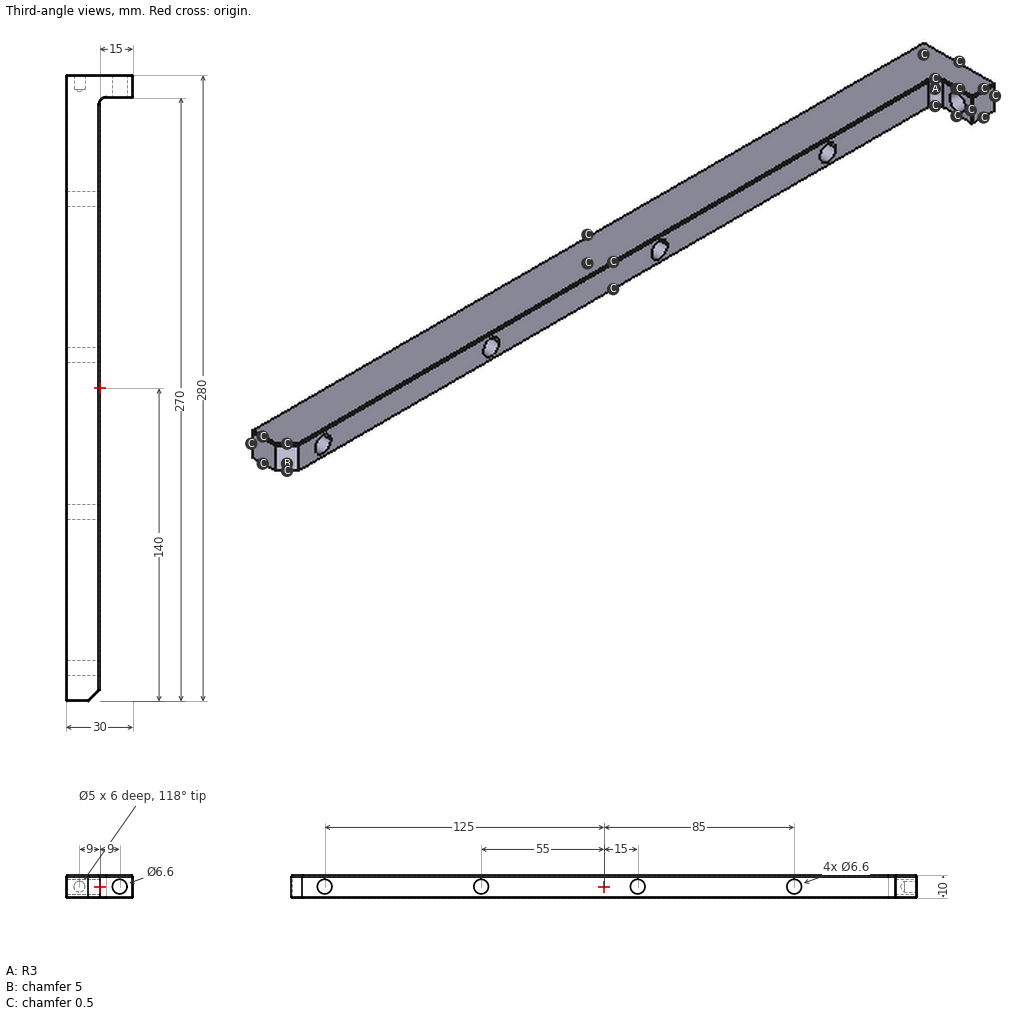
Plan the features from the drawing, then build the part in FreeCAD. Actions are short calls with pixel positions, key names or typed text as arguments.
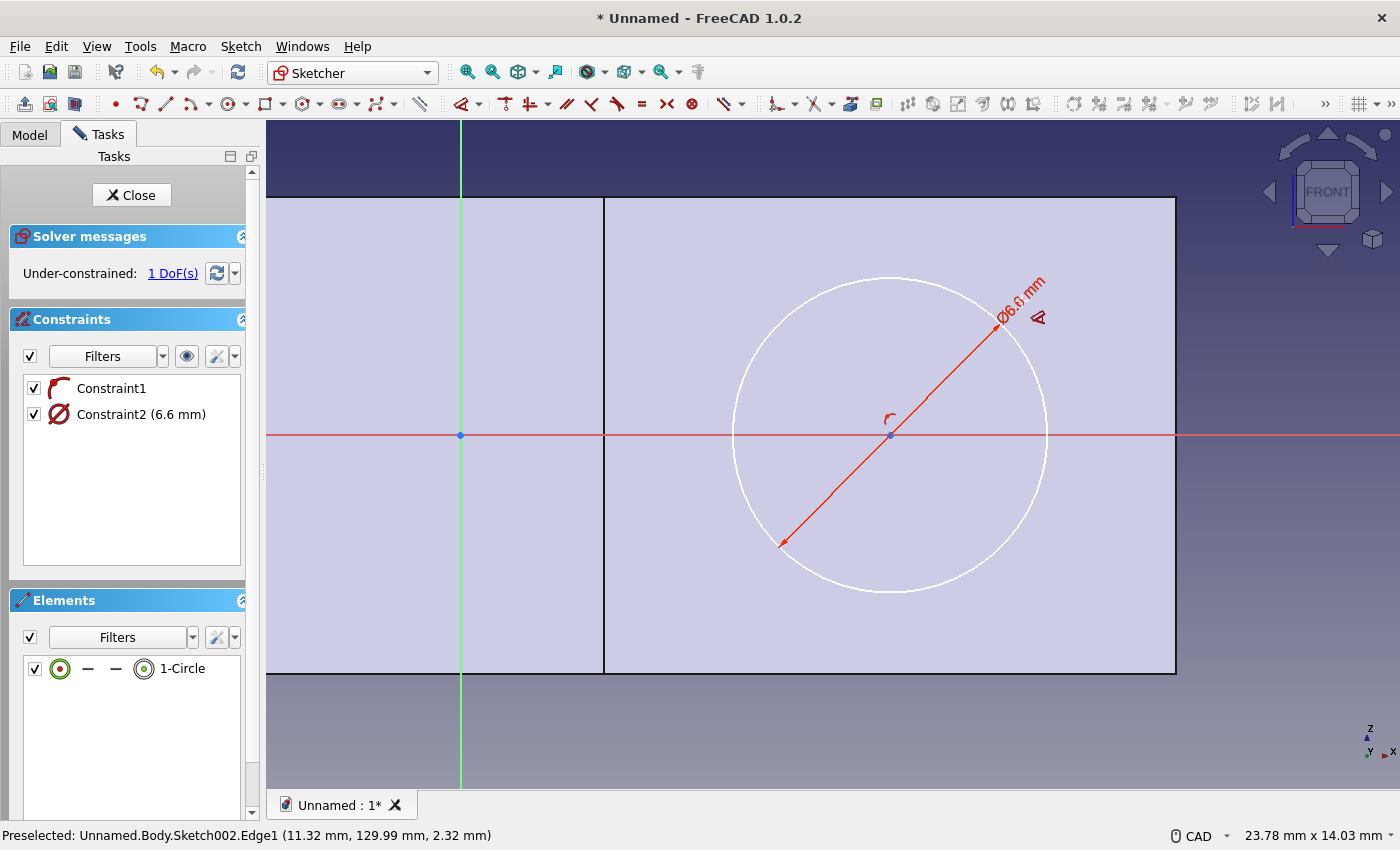
click(890, 435)
click(675, 469)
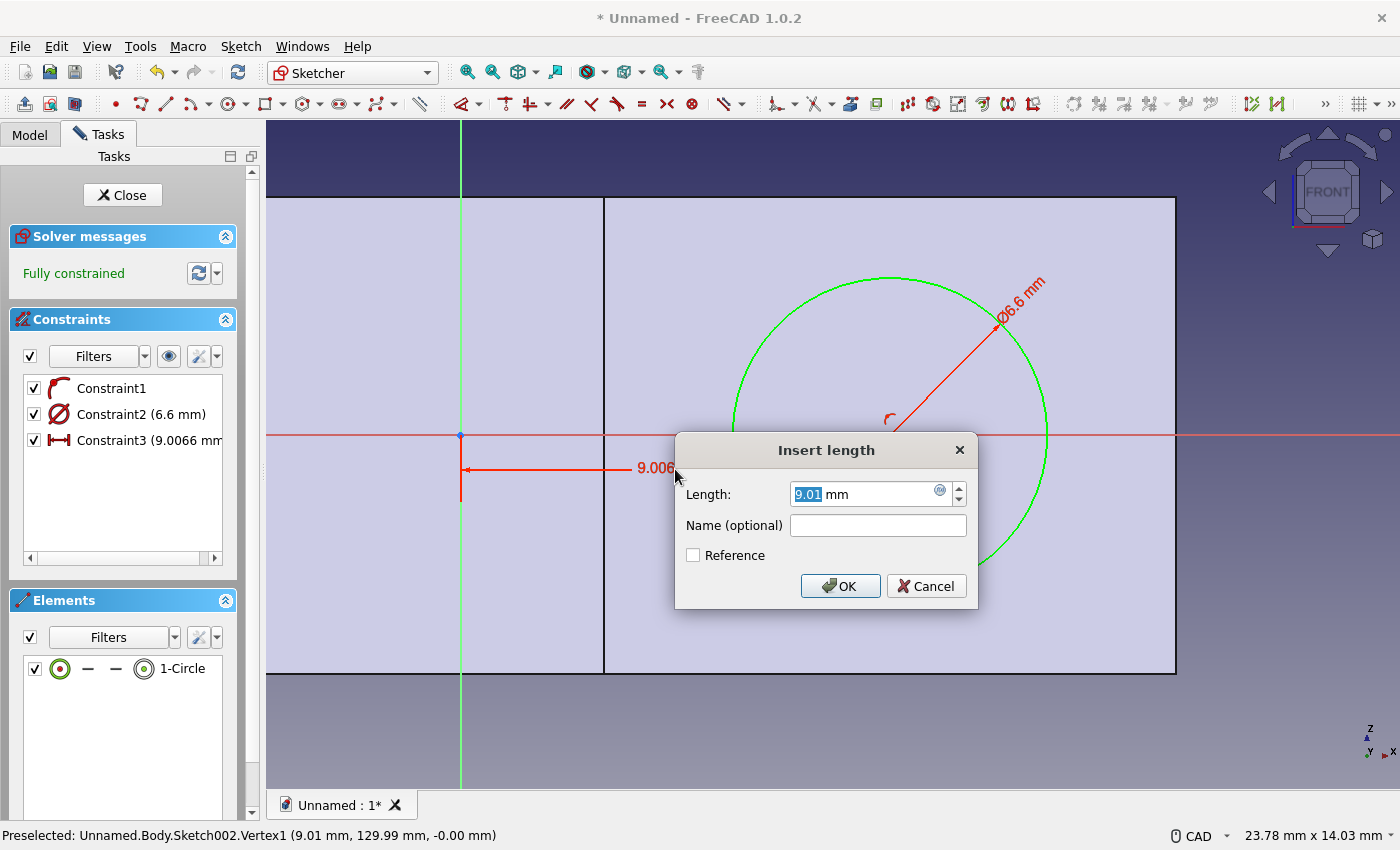
text(9)
key(Return)
key(Escape)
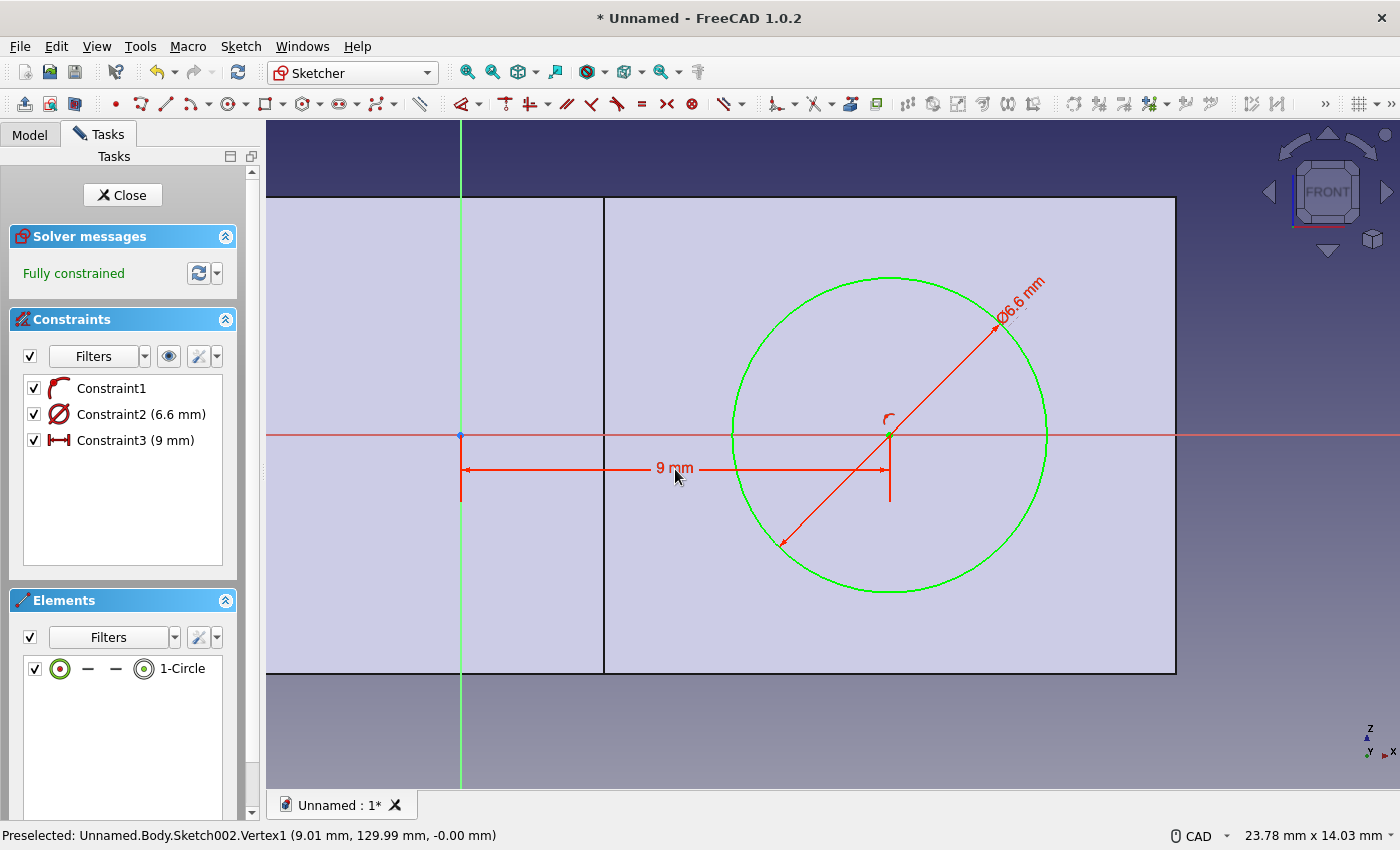
click(123, 195)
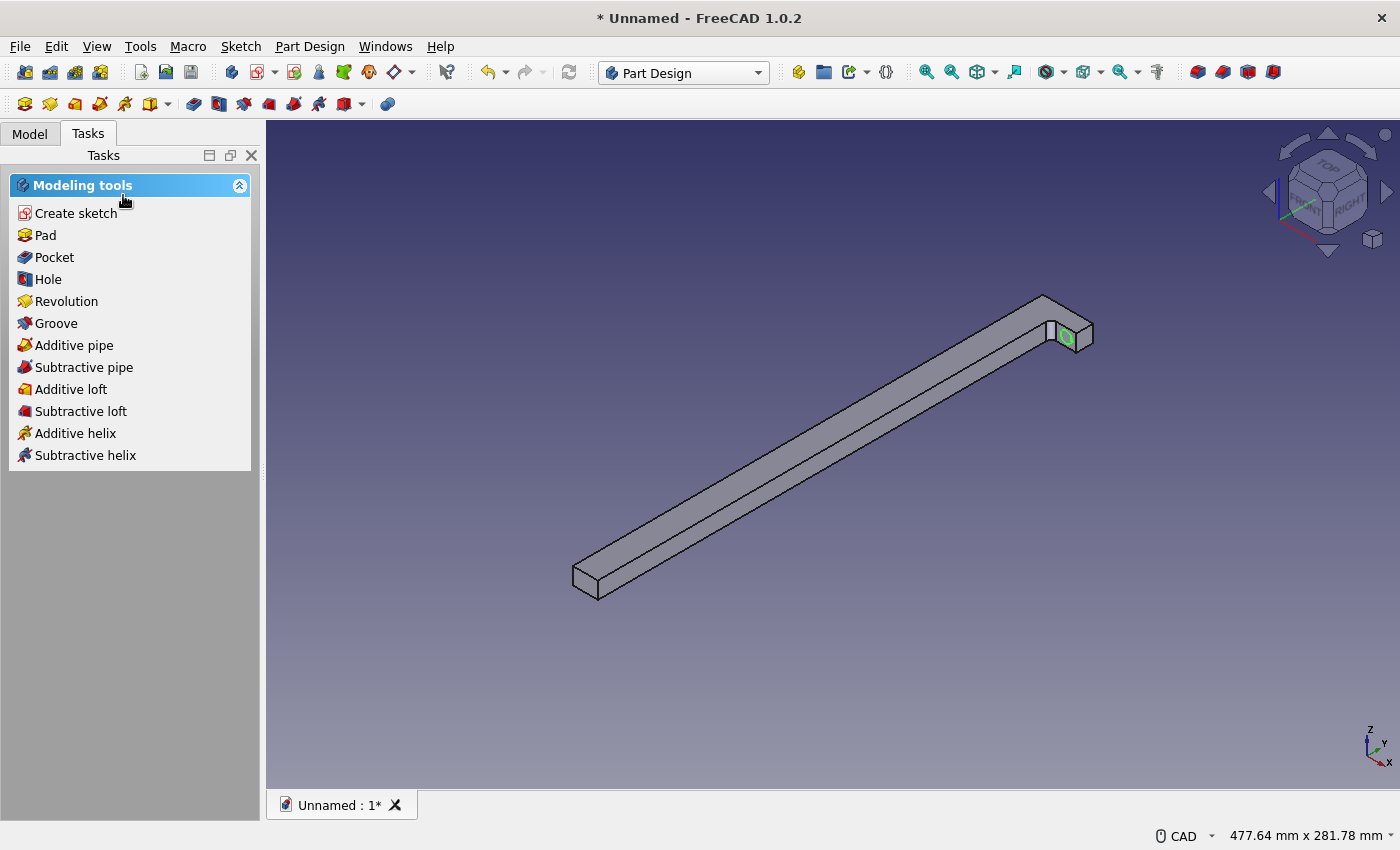
click(194, 104)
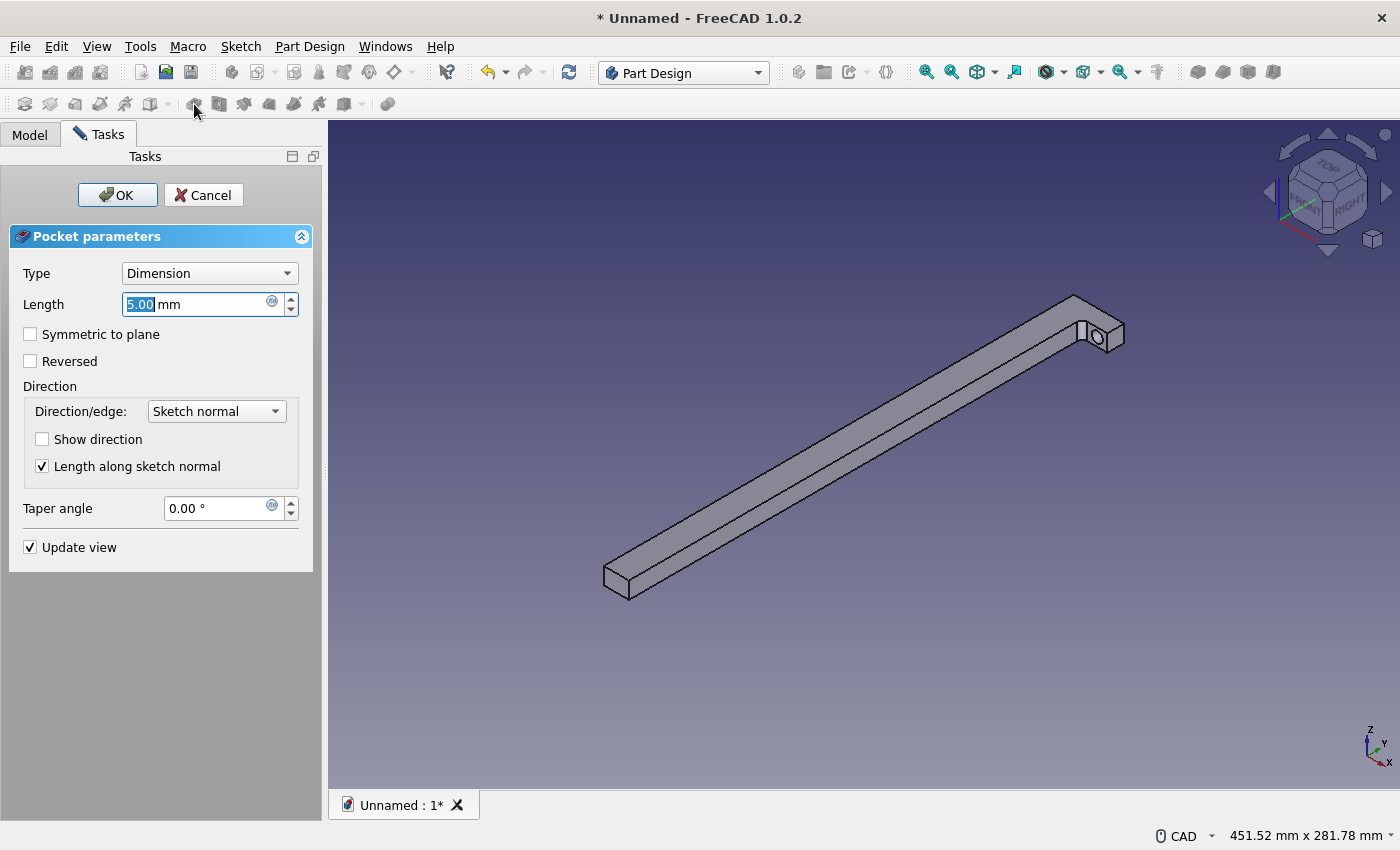
click(210, 274)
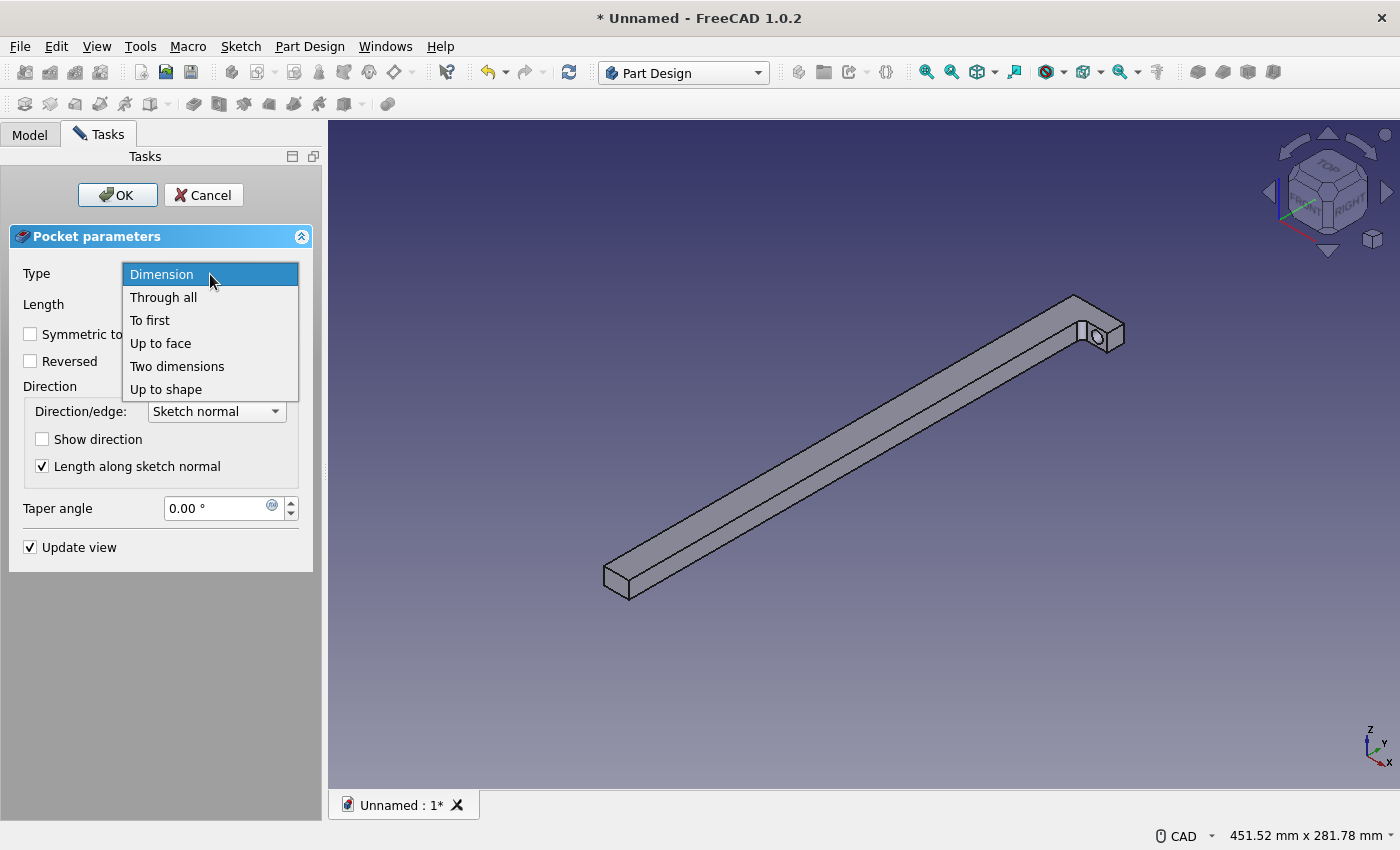
click(208, 298)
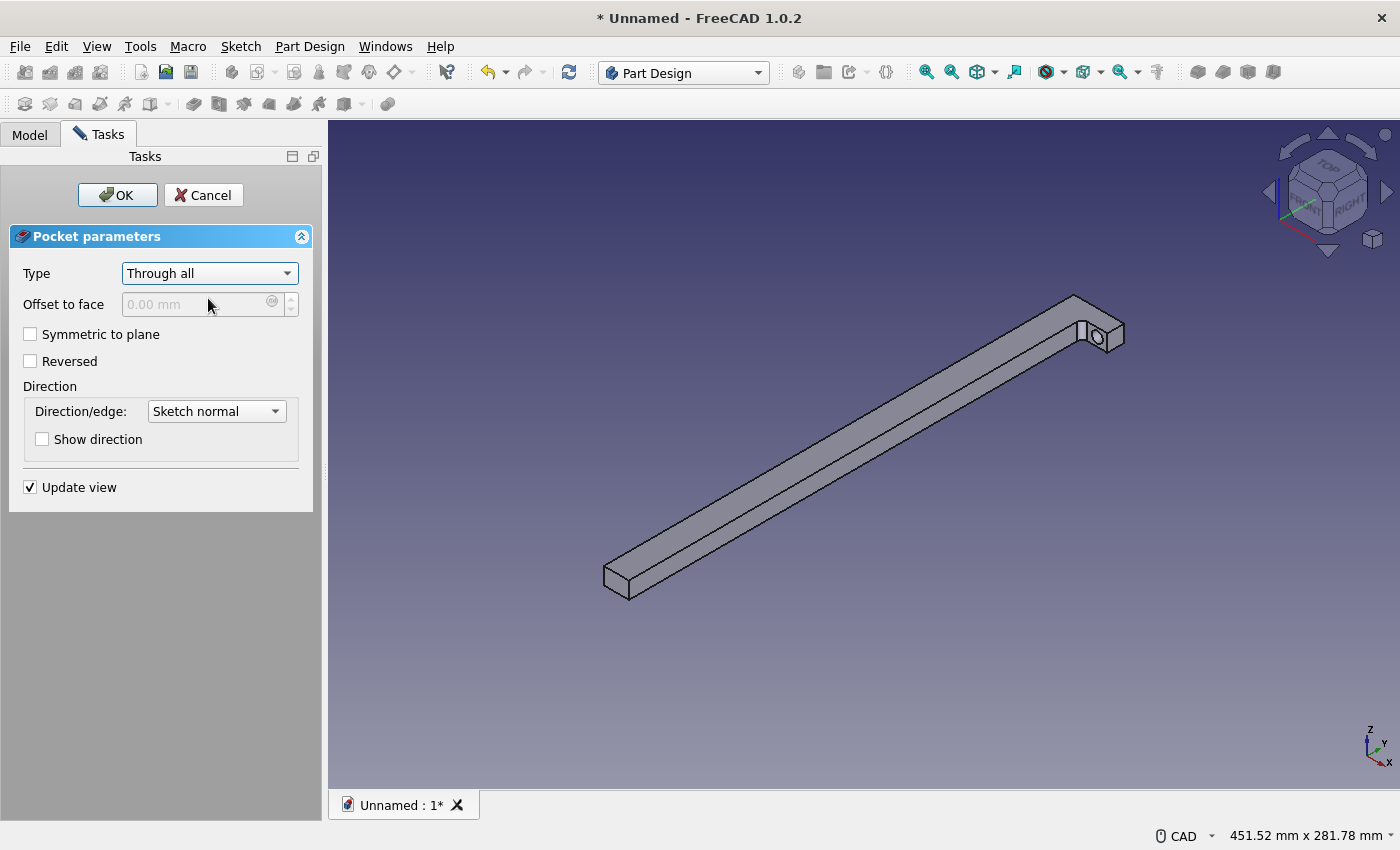
click(118, 195)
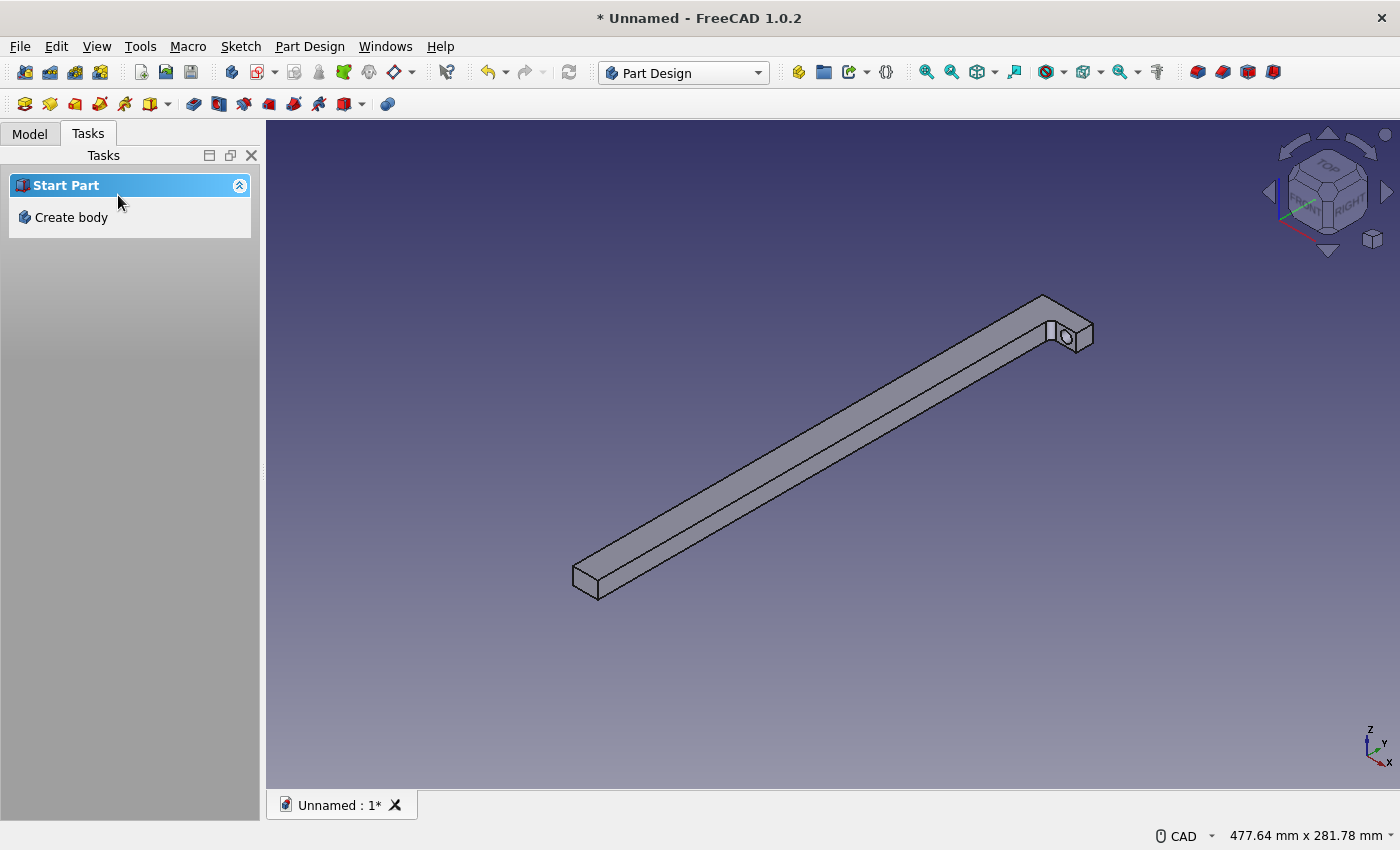
click(598, 589)